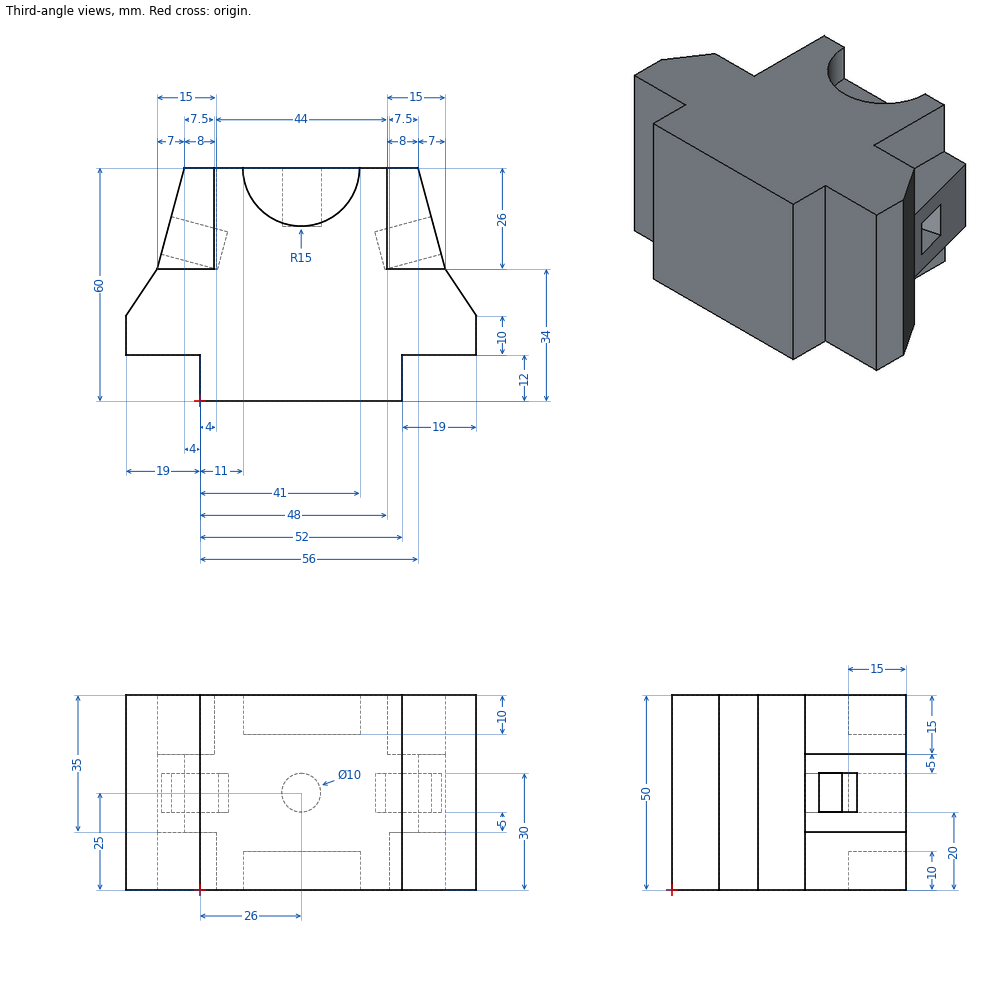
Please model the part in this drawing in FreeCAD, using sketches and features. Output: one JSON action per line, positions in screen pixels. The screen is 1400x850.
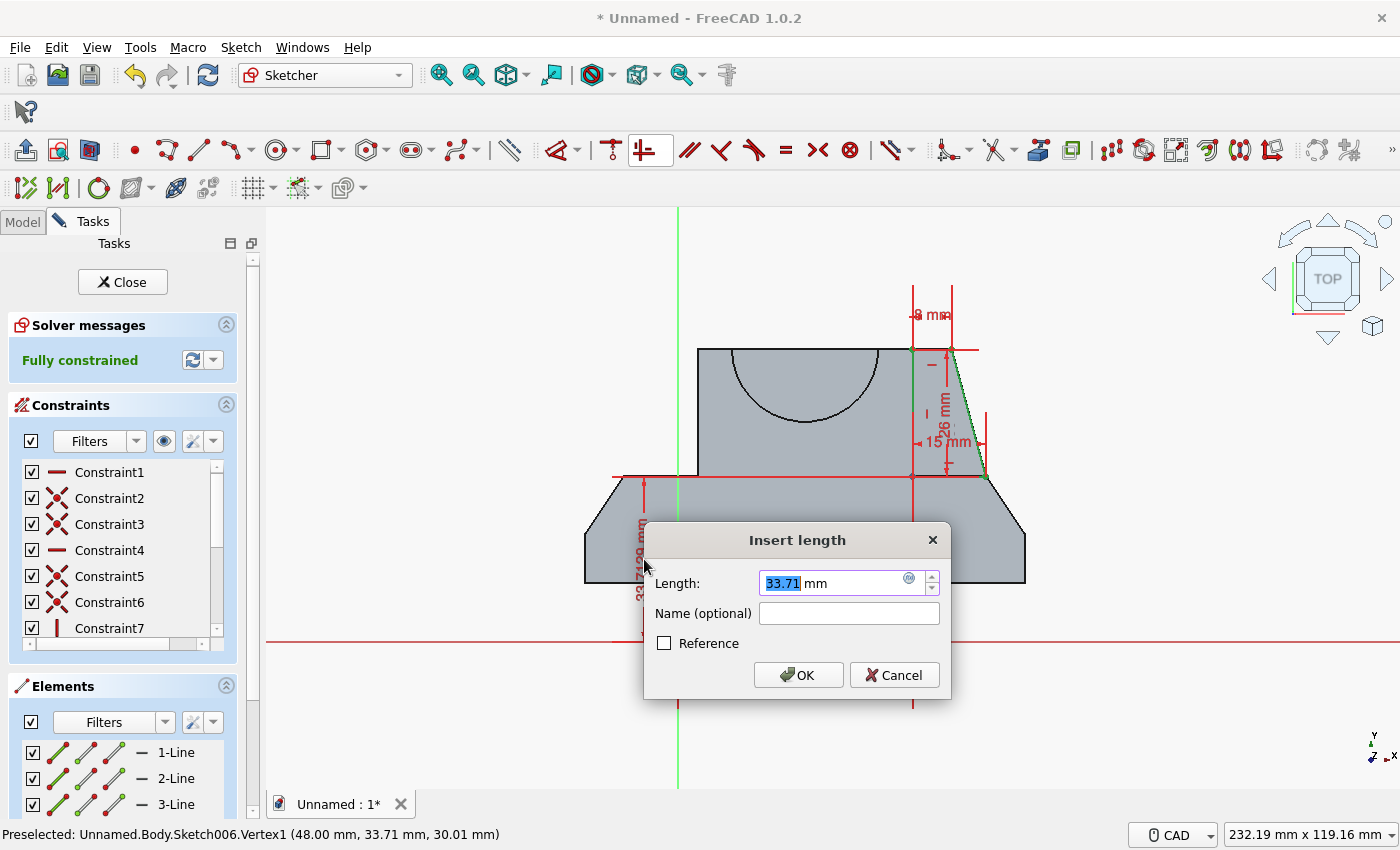
{"action": "type", "text": "34"}
{"action": "key", "text": "Return"}
{"action": "key", "text": "Escape"}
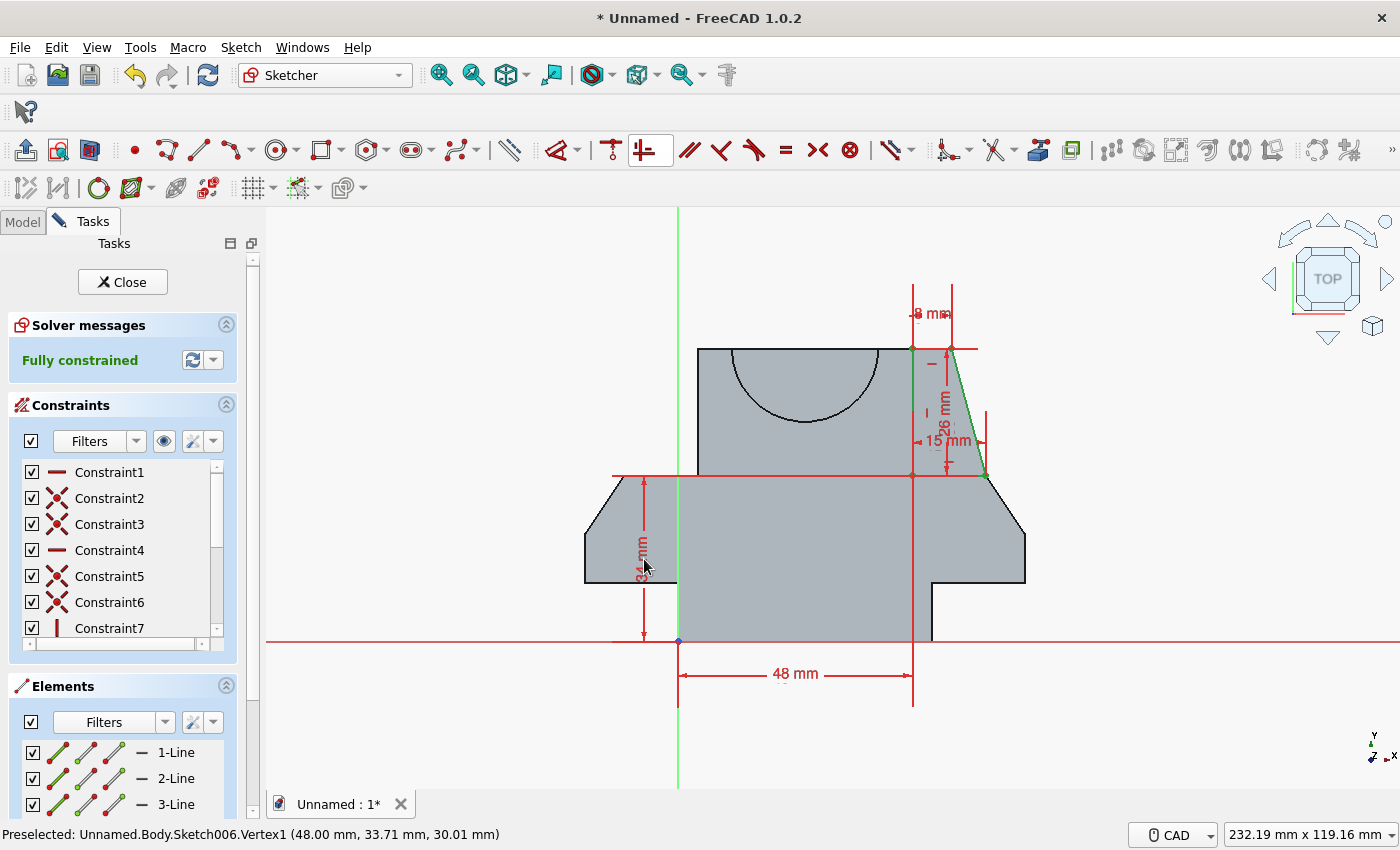
{"action": "left_click", "coordinate": [123, 282]}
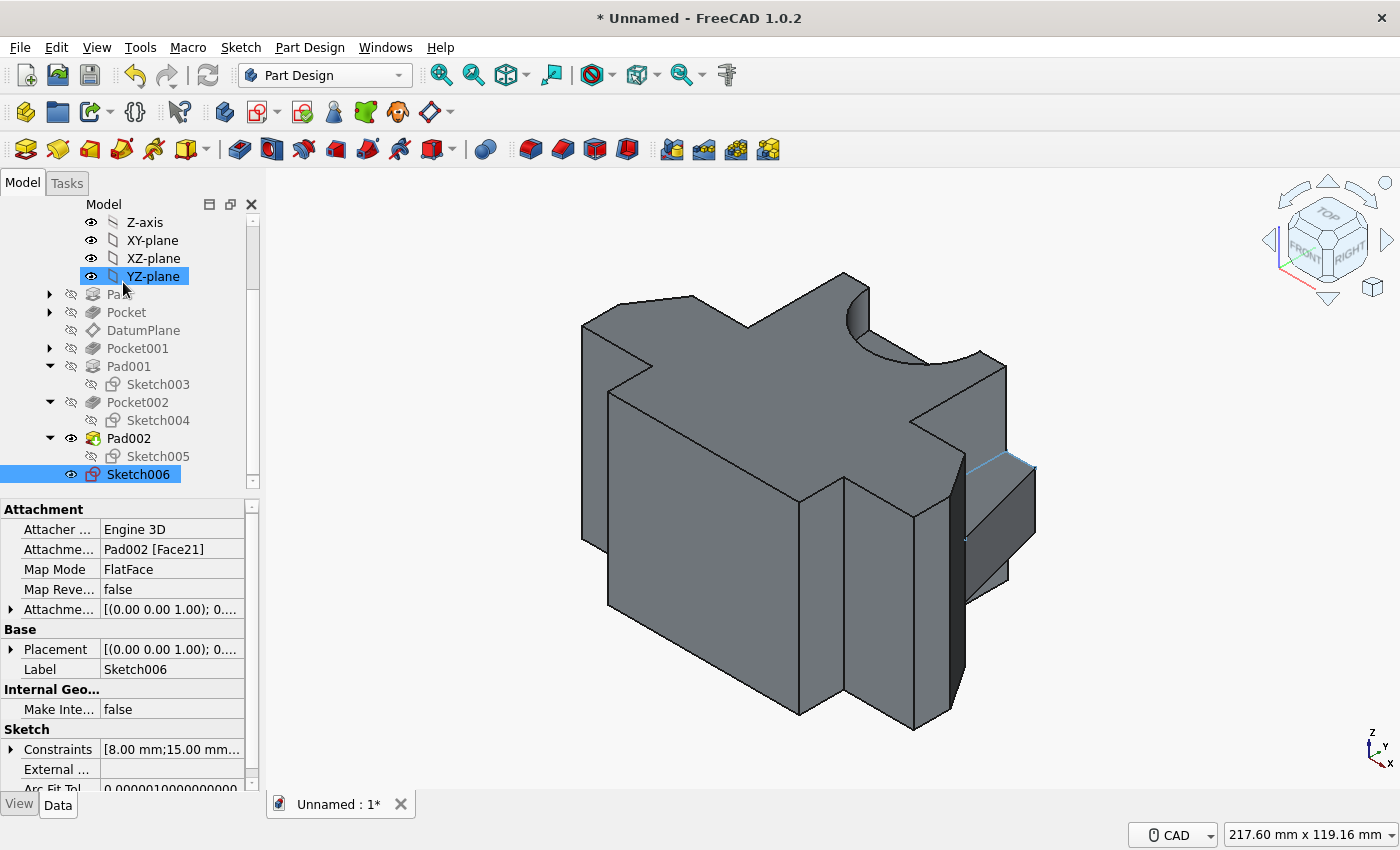
{"action": "left_click", "coordinate": [26, 150]}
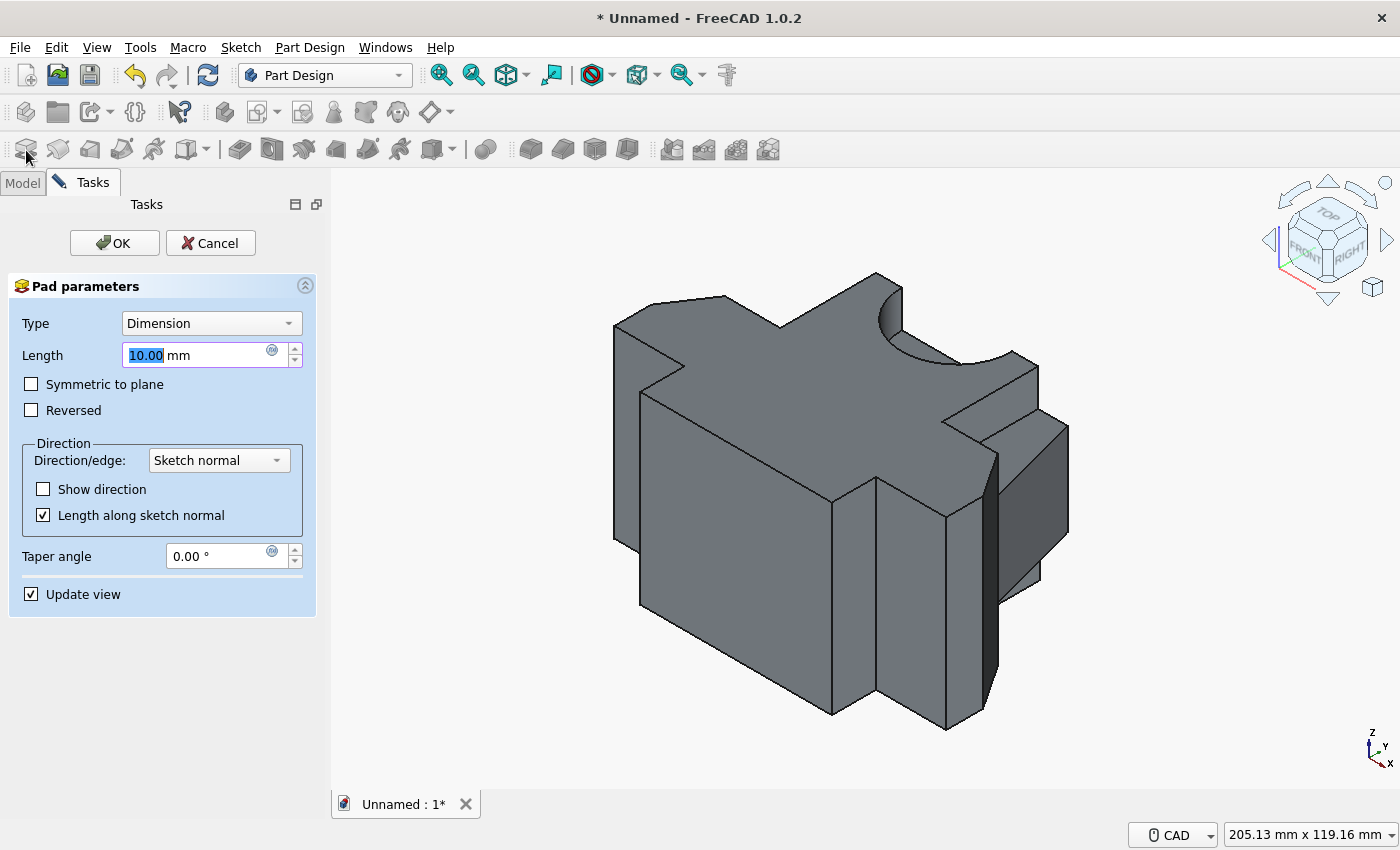
{"action": "type", "text": "5"}
{"action": "key", "text": "Tab"}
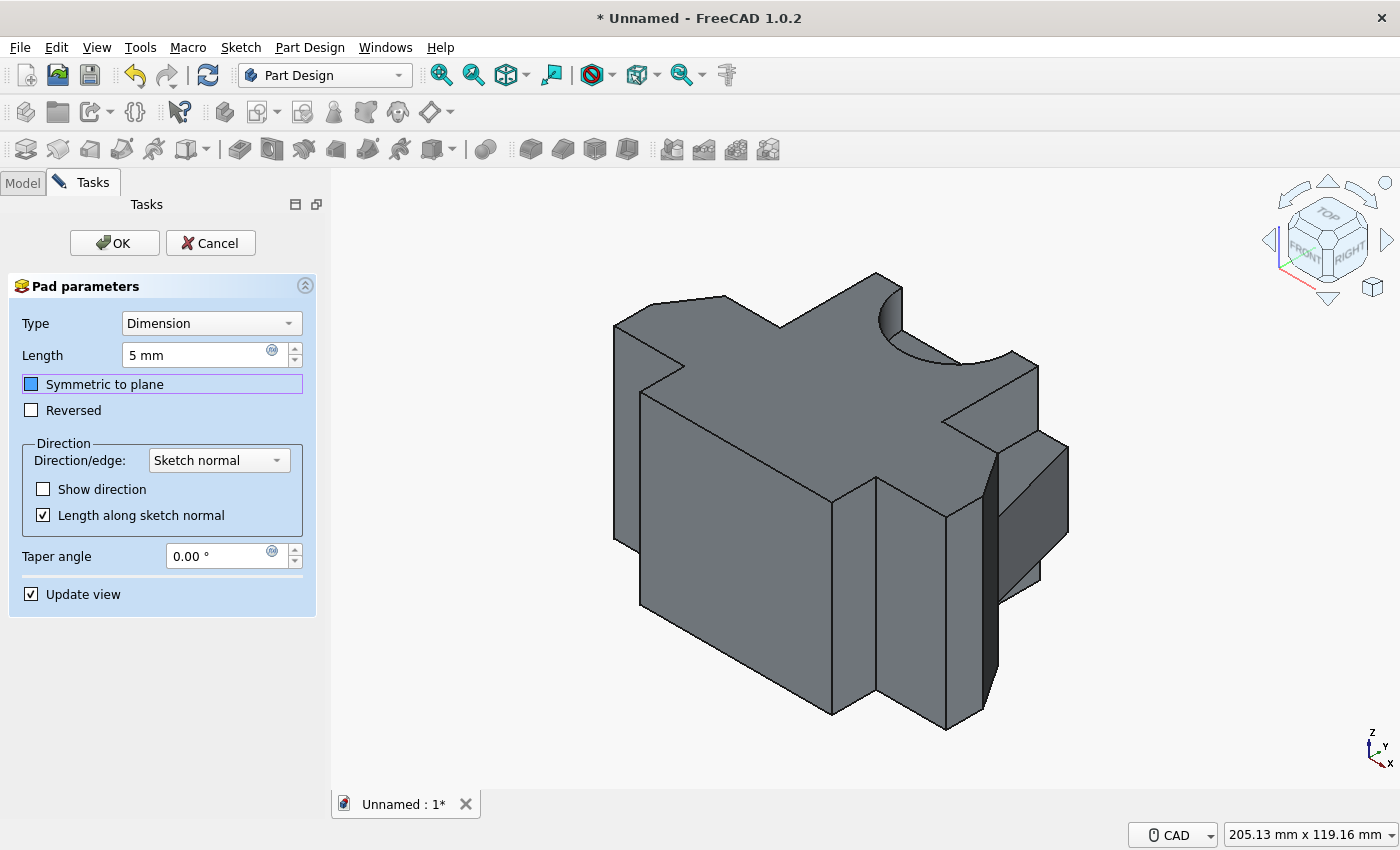
{"action": "left_click", "coordinate": [115, 243]}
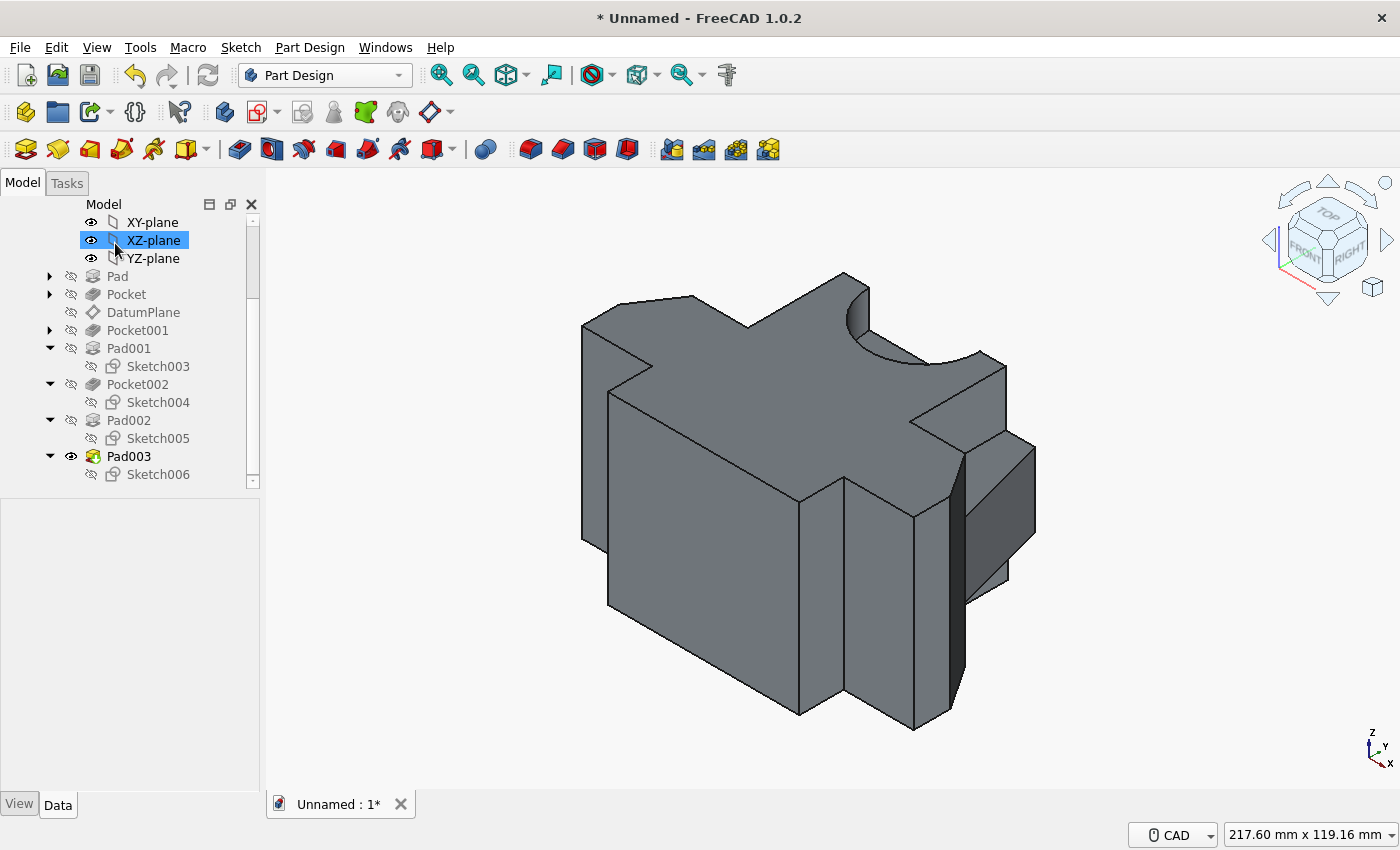
{"action": "left_click", "coordinate": [783, 401]}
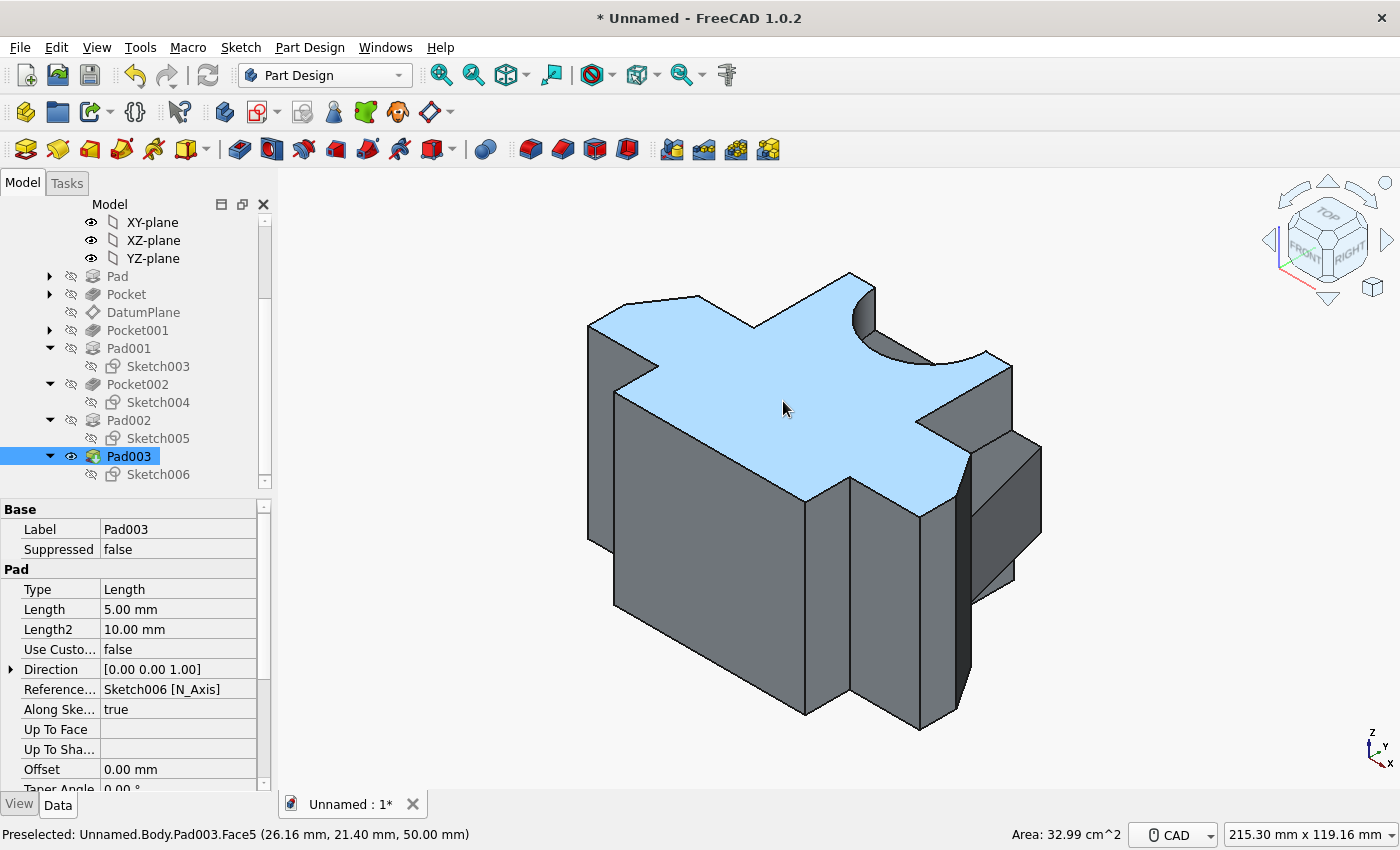
{"action": "left_click", "coordinate": [258, 112]}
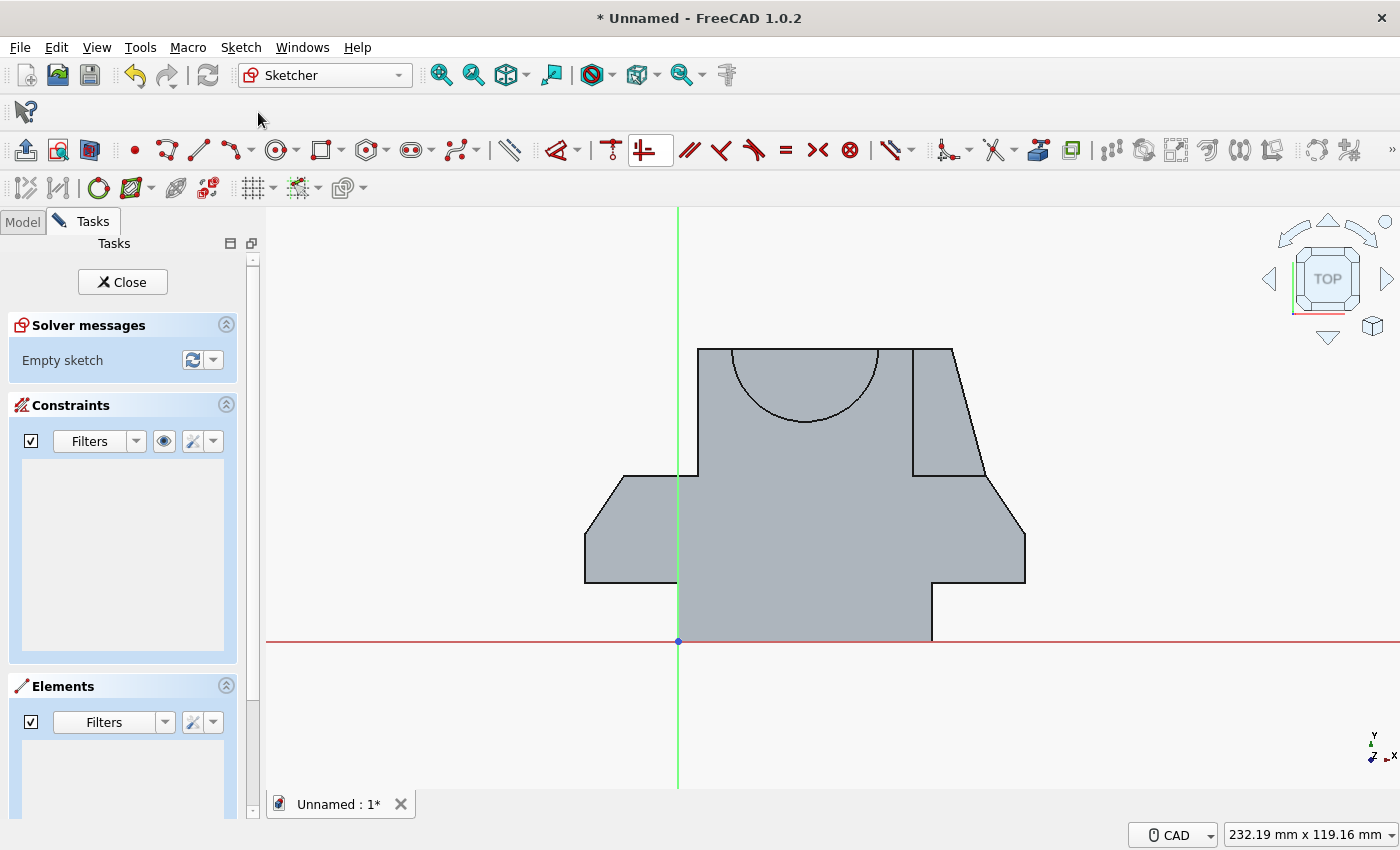
{"action": "left_click", "coordinate": [168, 150]}